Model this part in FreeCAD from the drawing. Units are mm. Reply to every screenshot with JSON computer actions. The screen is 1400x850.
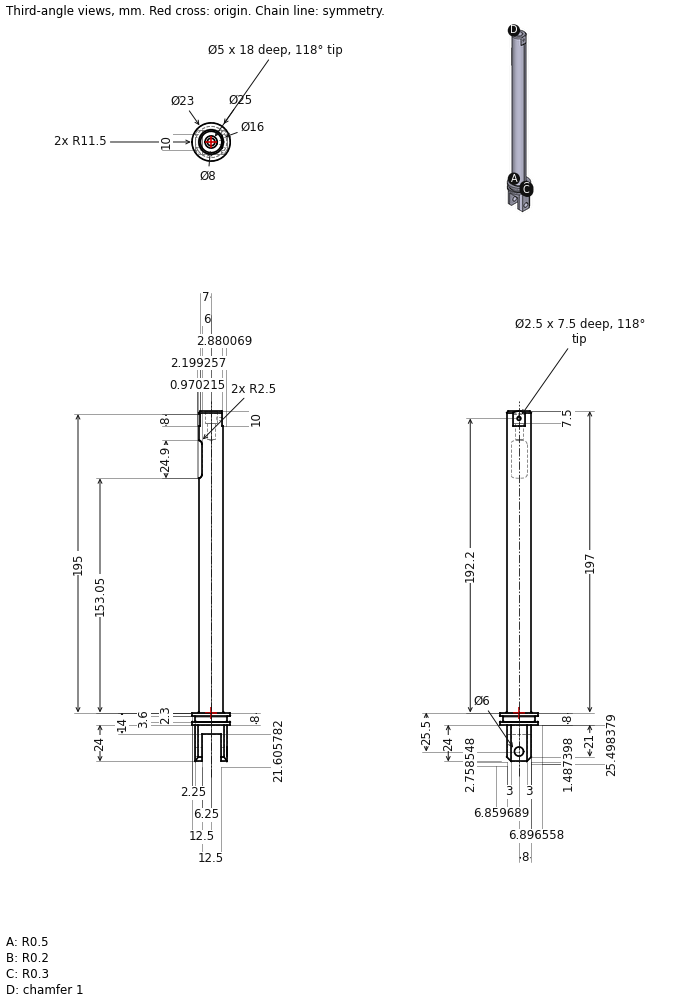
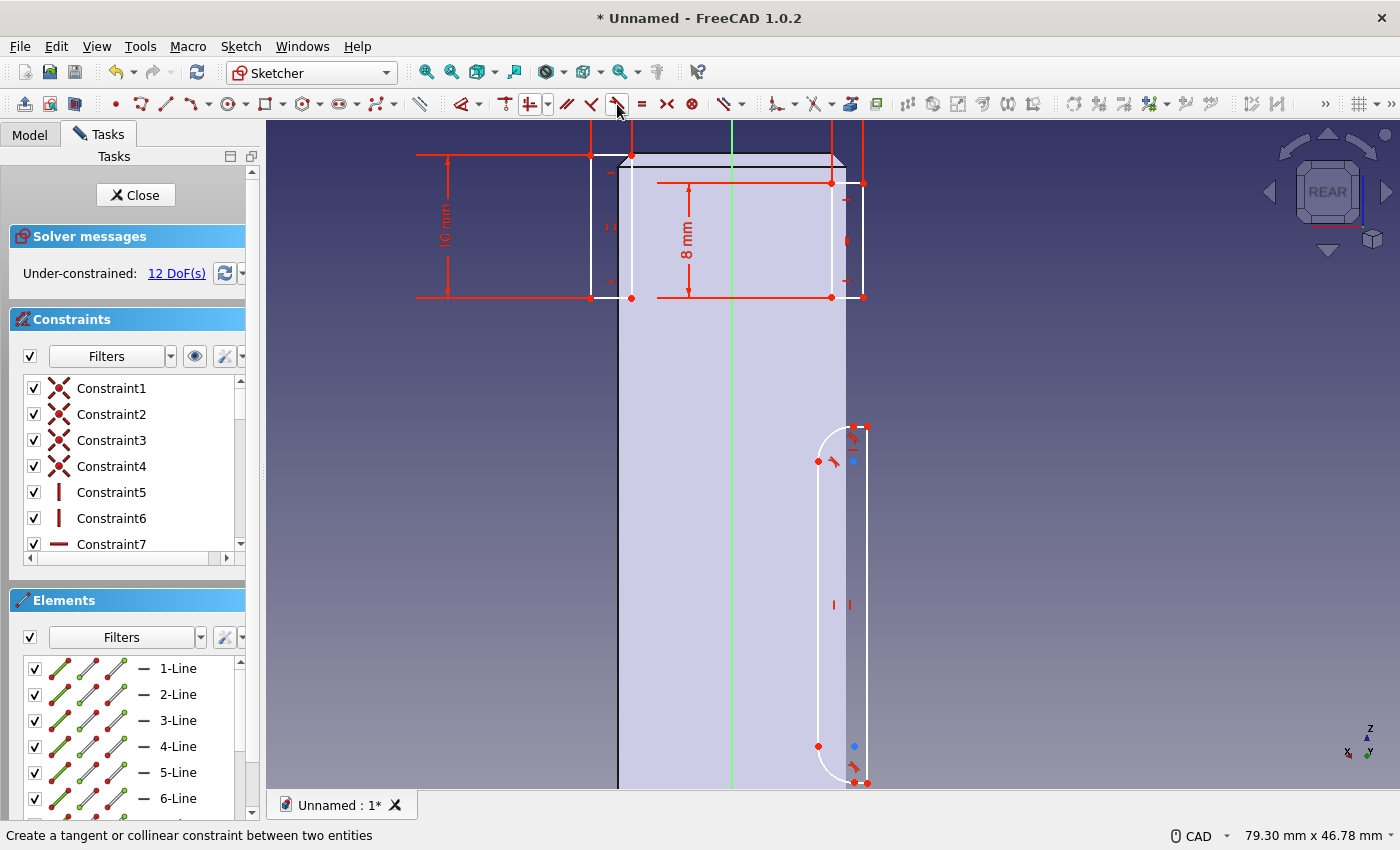
{"action": "left_click", "coordinate": [818, 547]}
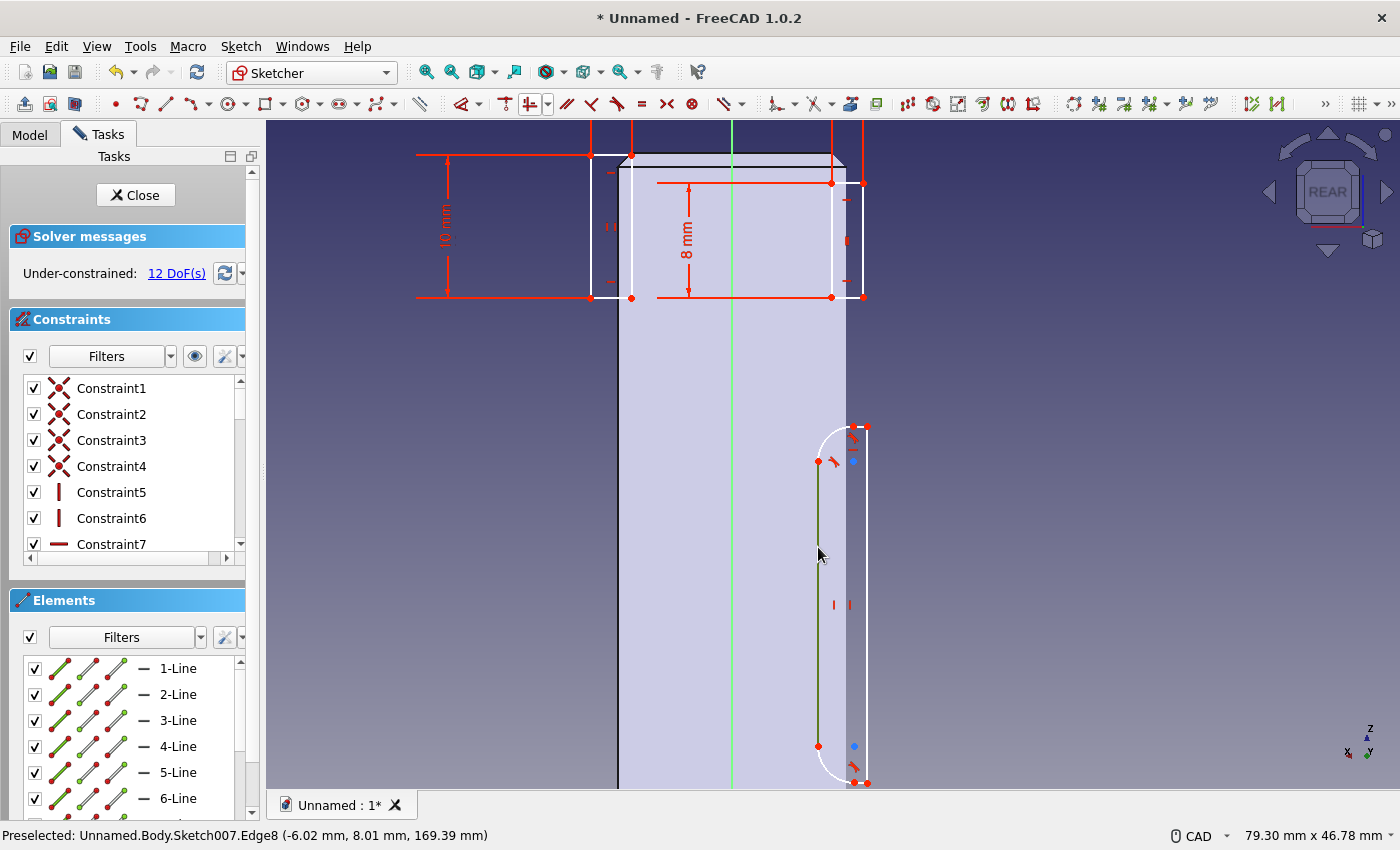
{"action": "scroll", "coordinate": [820, 758], "scroll_direction": "up", "scroll_amount": 2}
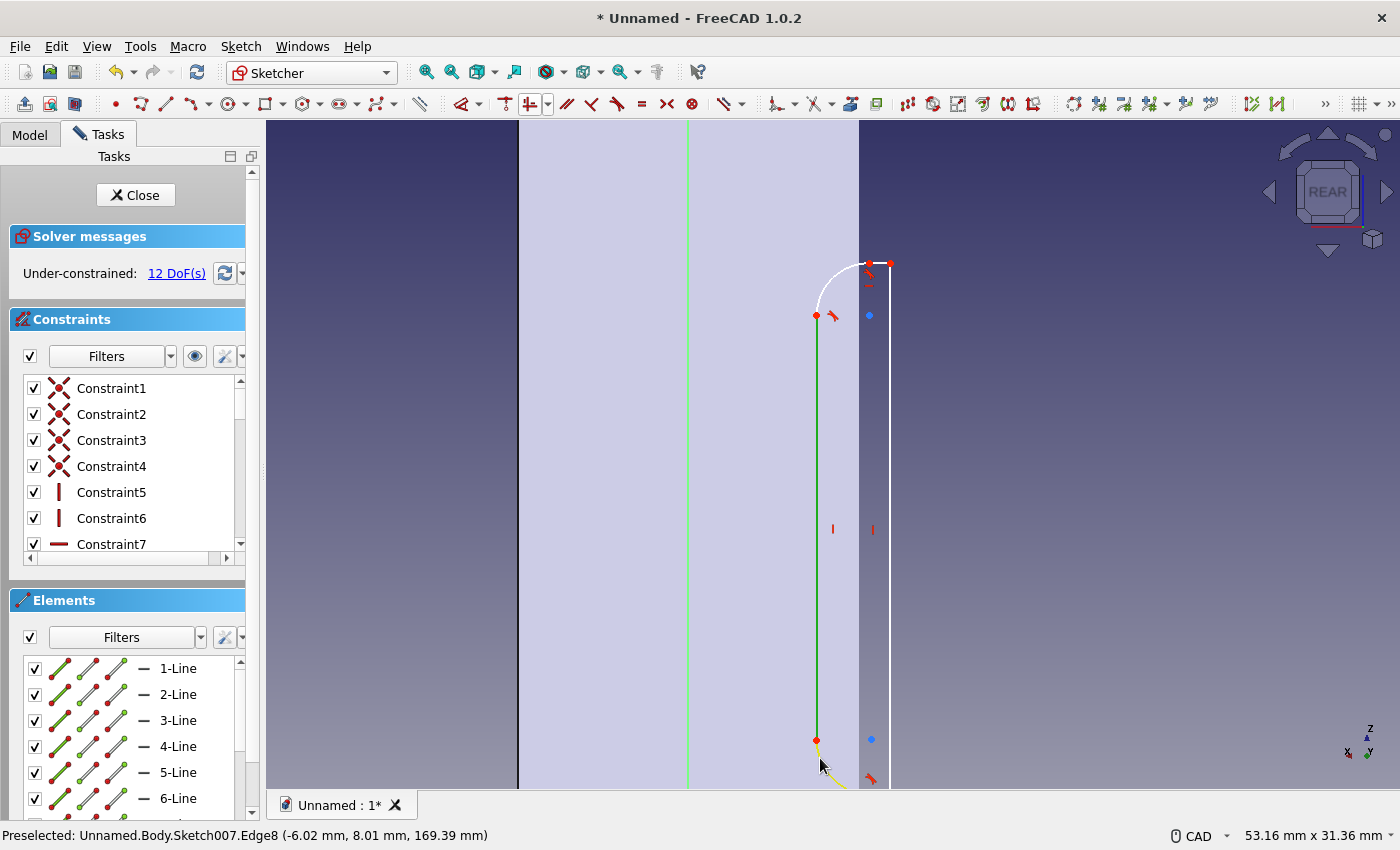
{"action": "left_click", "coordinate": [820, 757]}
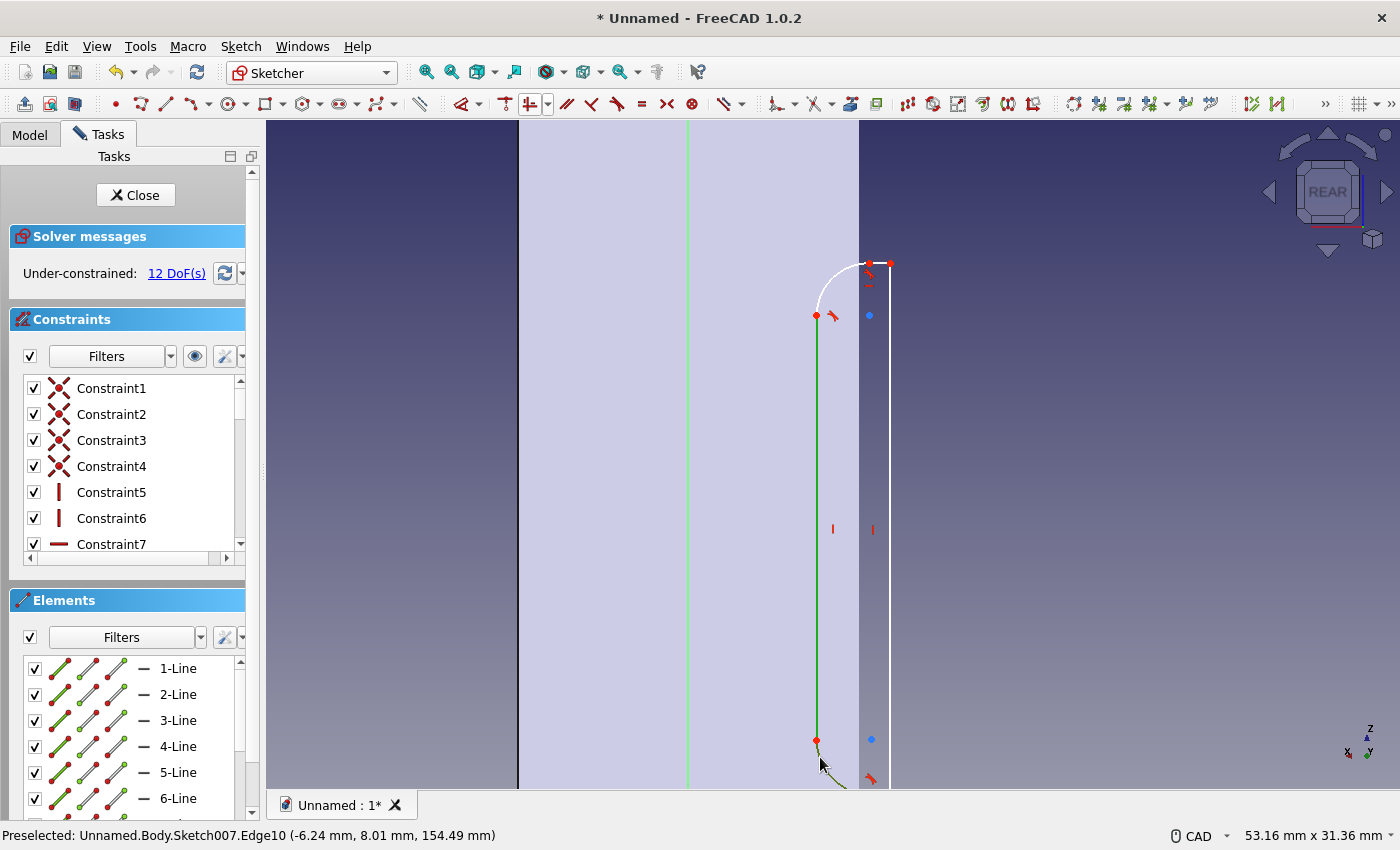
{"action": "left_click", "coordinate": [617, 104]}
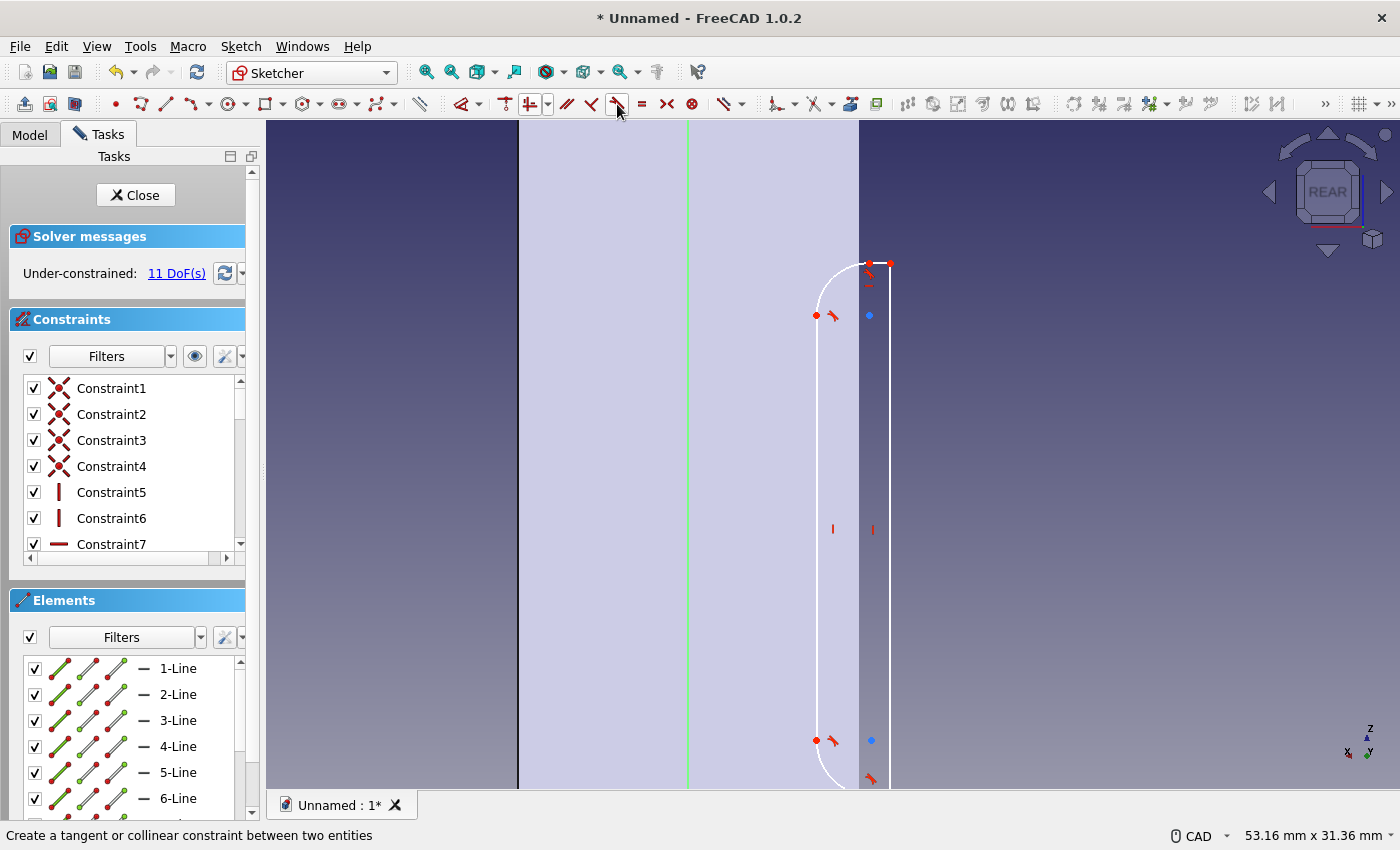
{"action": "scroll", "coordinate": [830, 561], "scroll_direction": "down", "scroll_amount": 4}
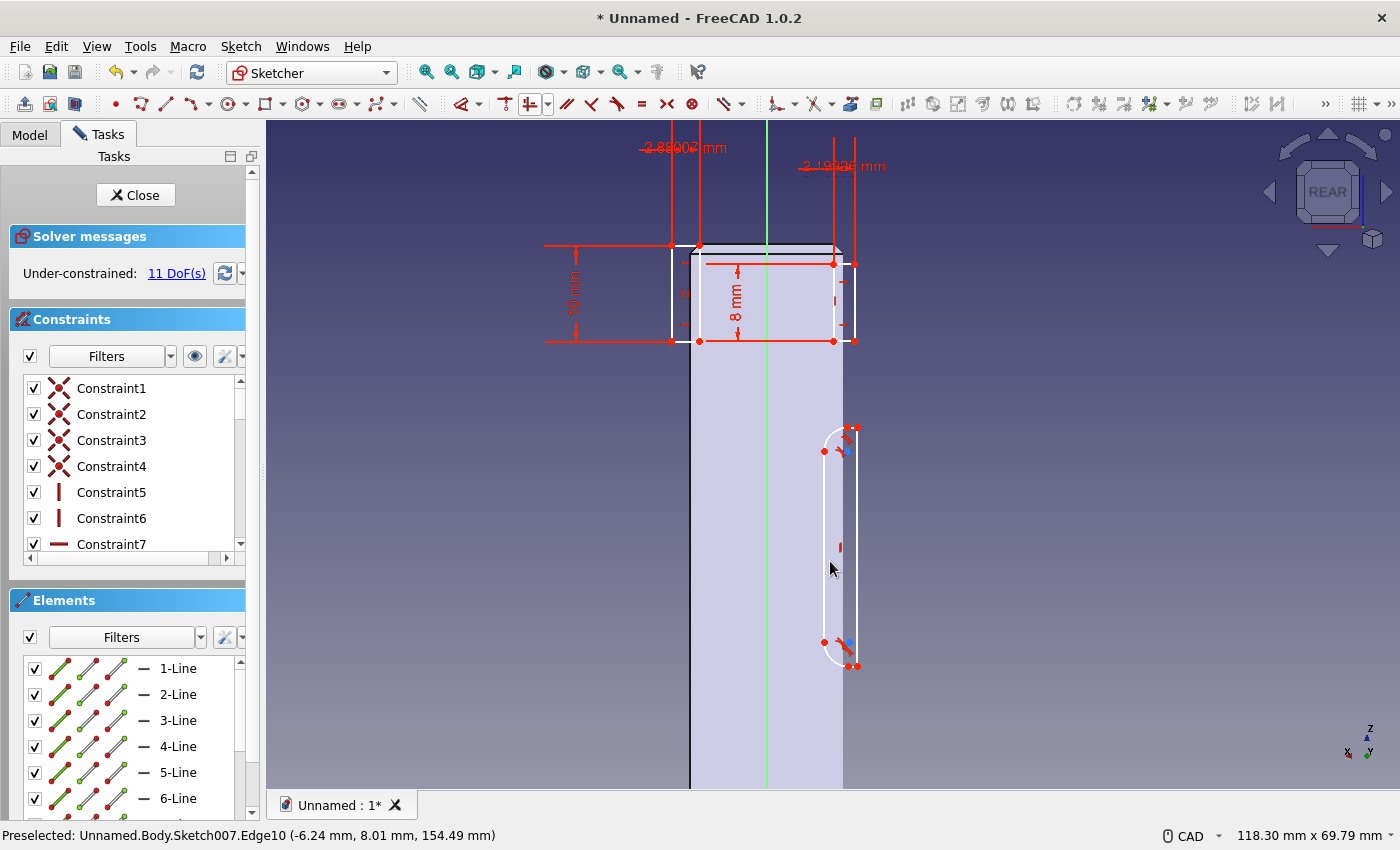
{"action": "scroll", "coordinate": [853, 667], "scroll_direction": "up", "scroll_amount": 6}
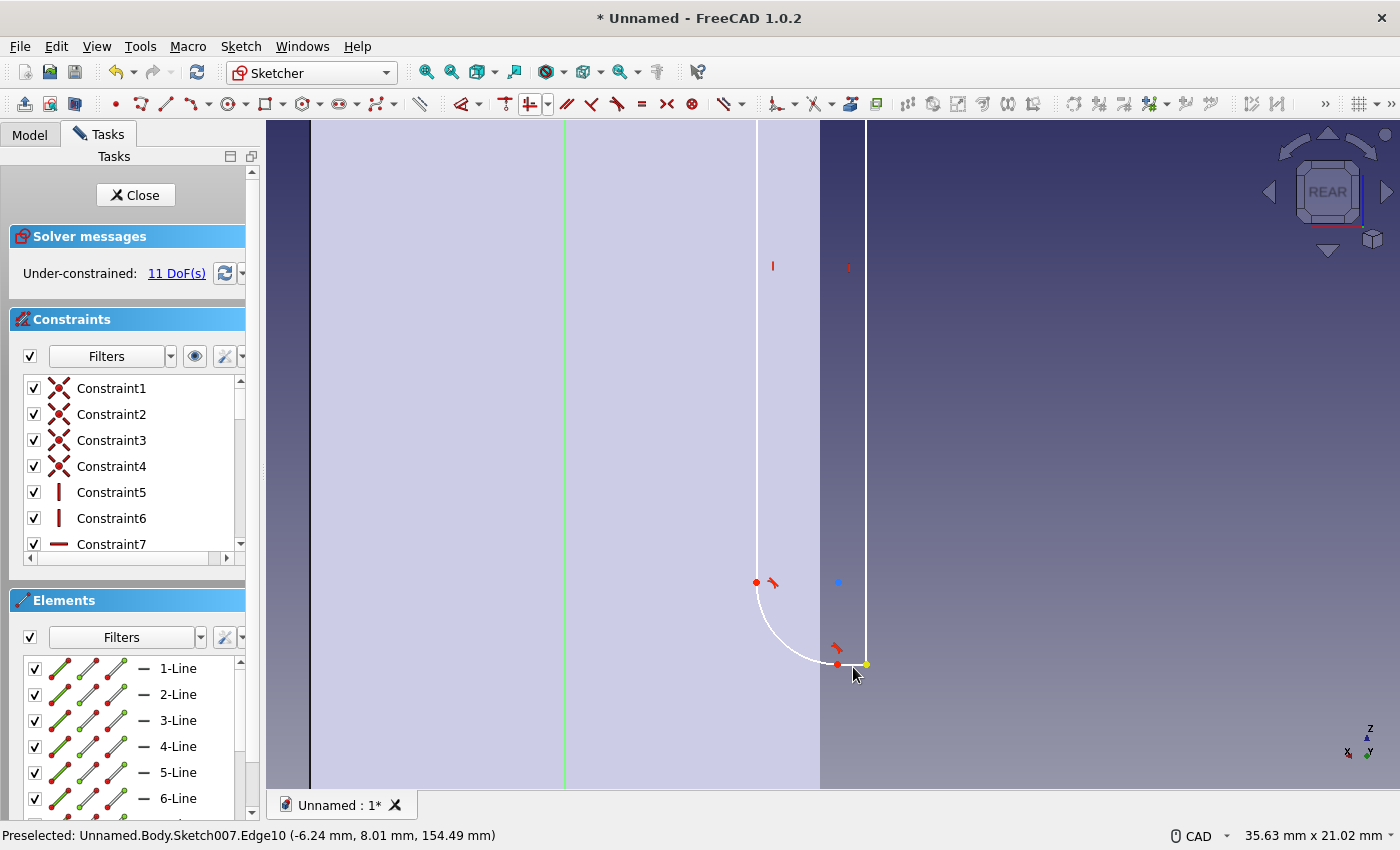
{"action": "left_click", "coordinate": [852, 665]}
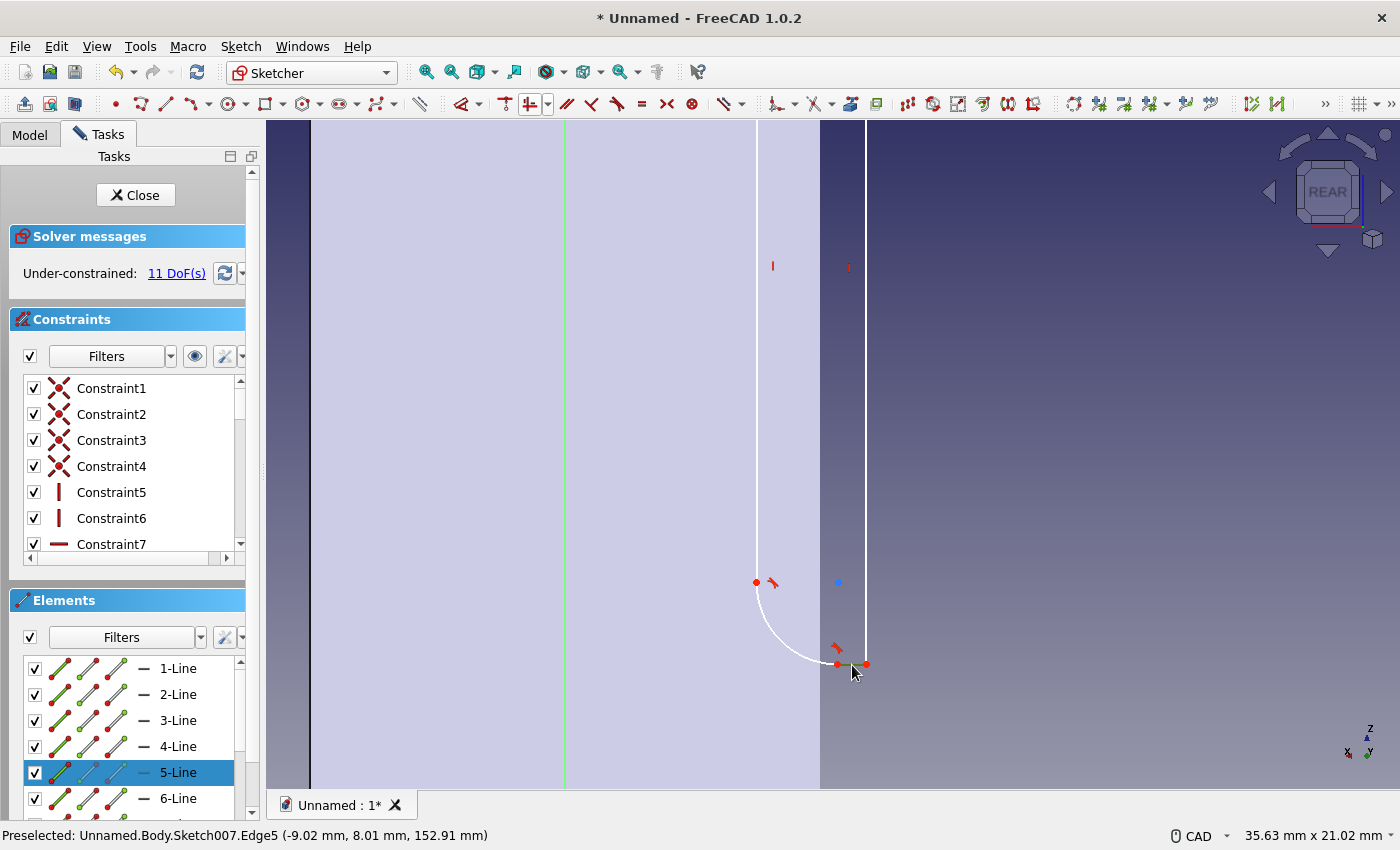
{"action": "left_click", "coordinate": [548, 104]}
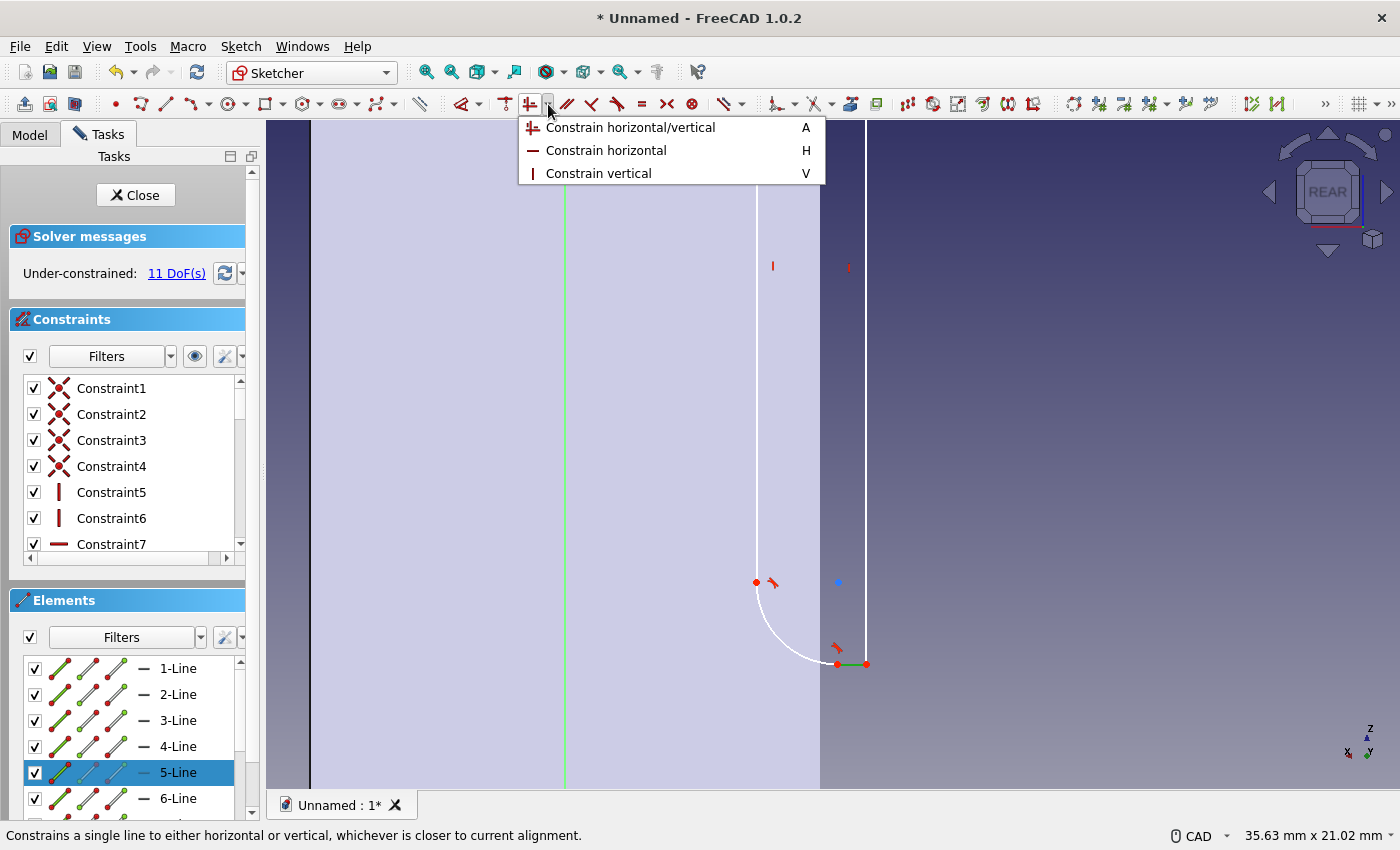
{"action": "left_click", "coordinate": [672, 150]}